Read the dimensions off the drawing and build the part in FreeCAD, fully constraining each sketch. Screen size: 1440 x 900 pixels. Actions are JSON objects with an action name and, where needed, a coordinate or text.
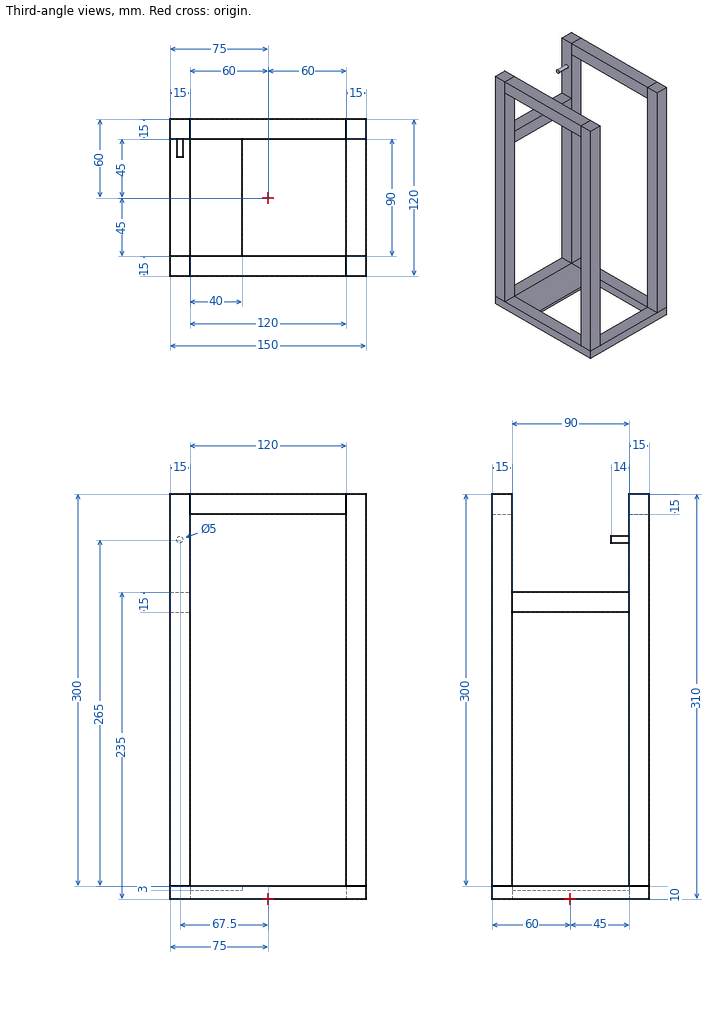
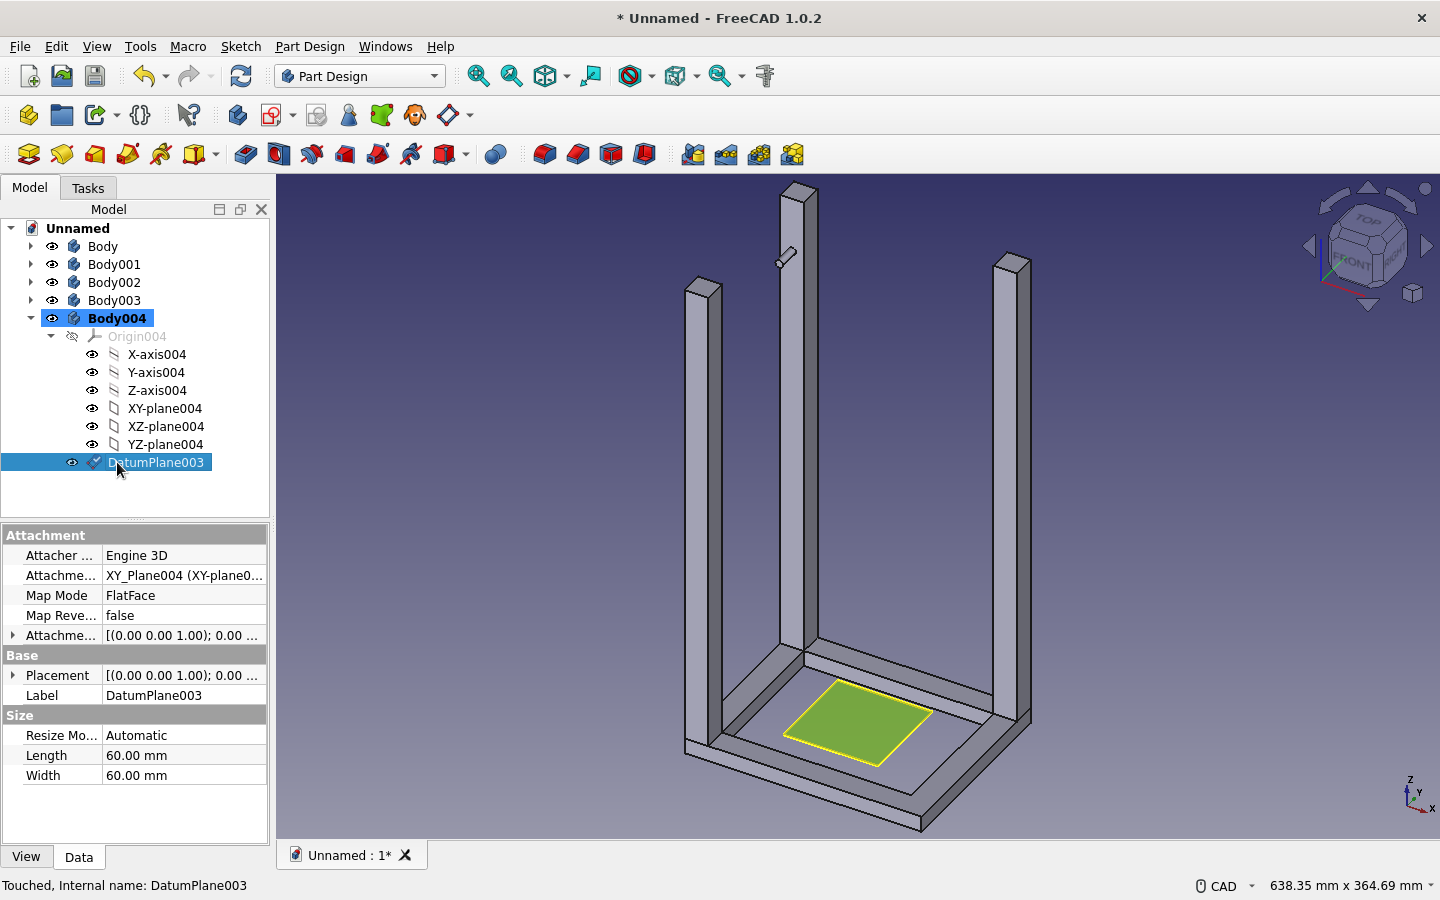
{"action": "left_click", "coordinate": [270, 116]}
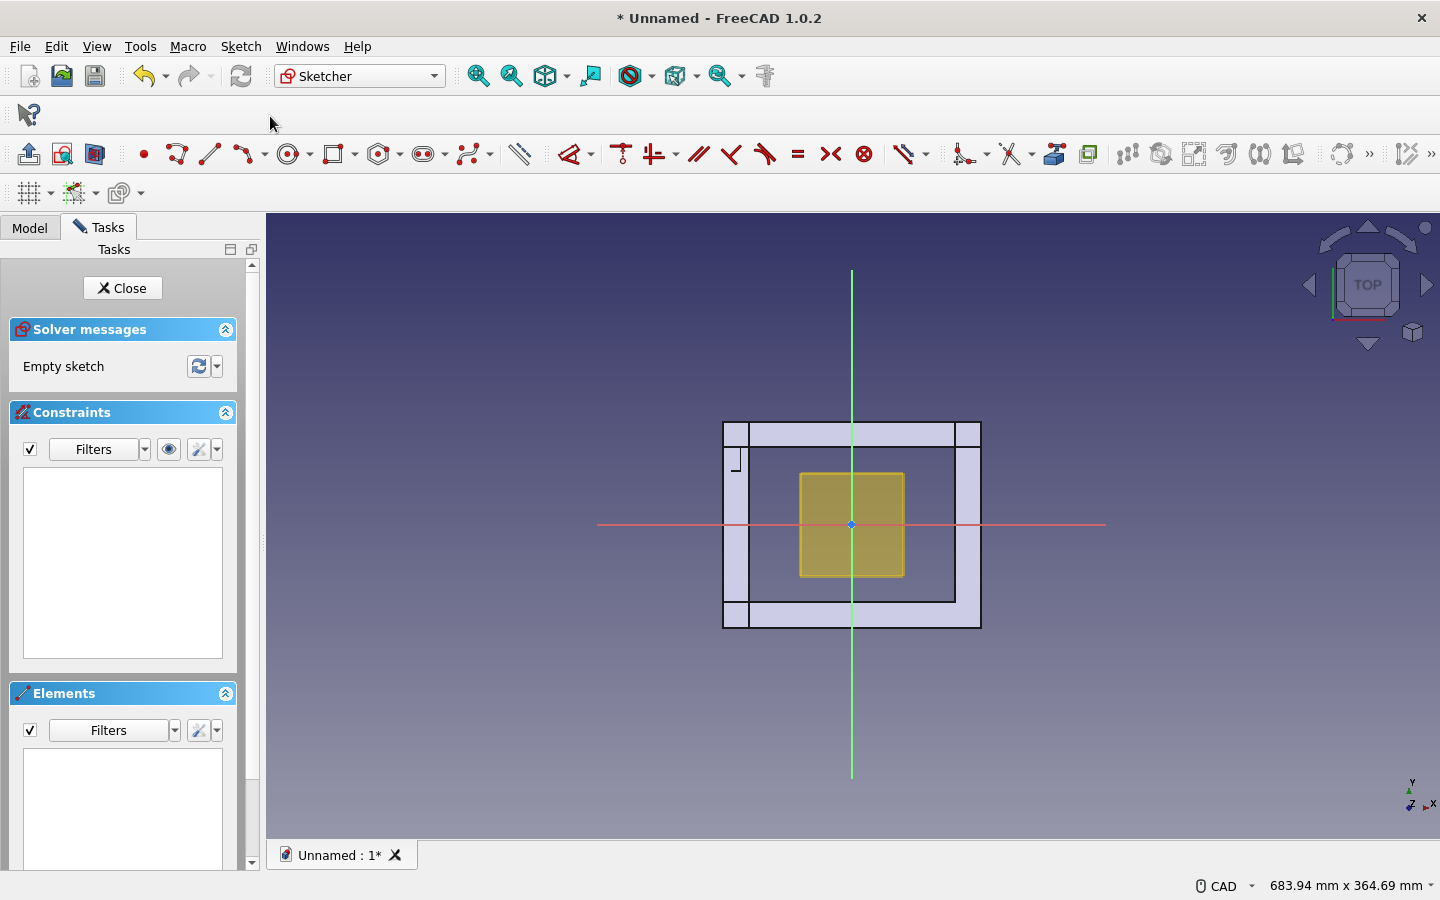
{"action": "scroll", "coordinate": [980, 620], "scroll_direction": "up", "scroll_amount": 14}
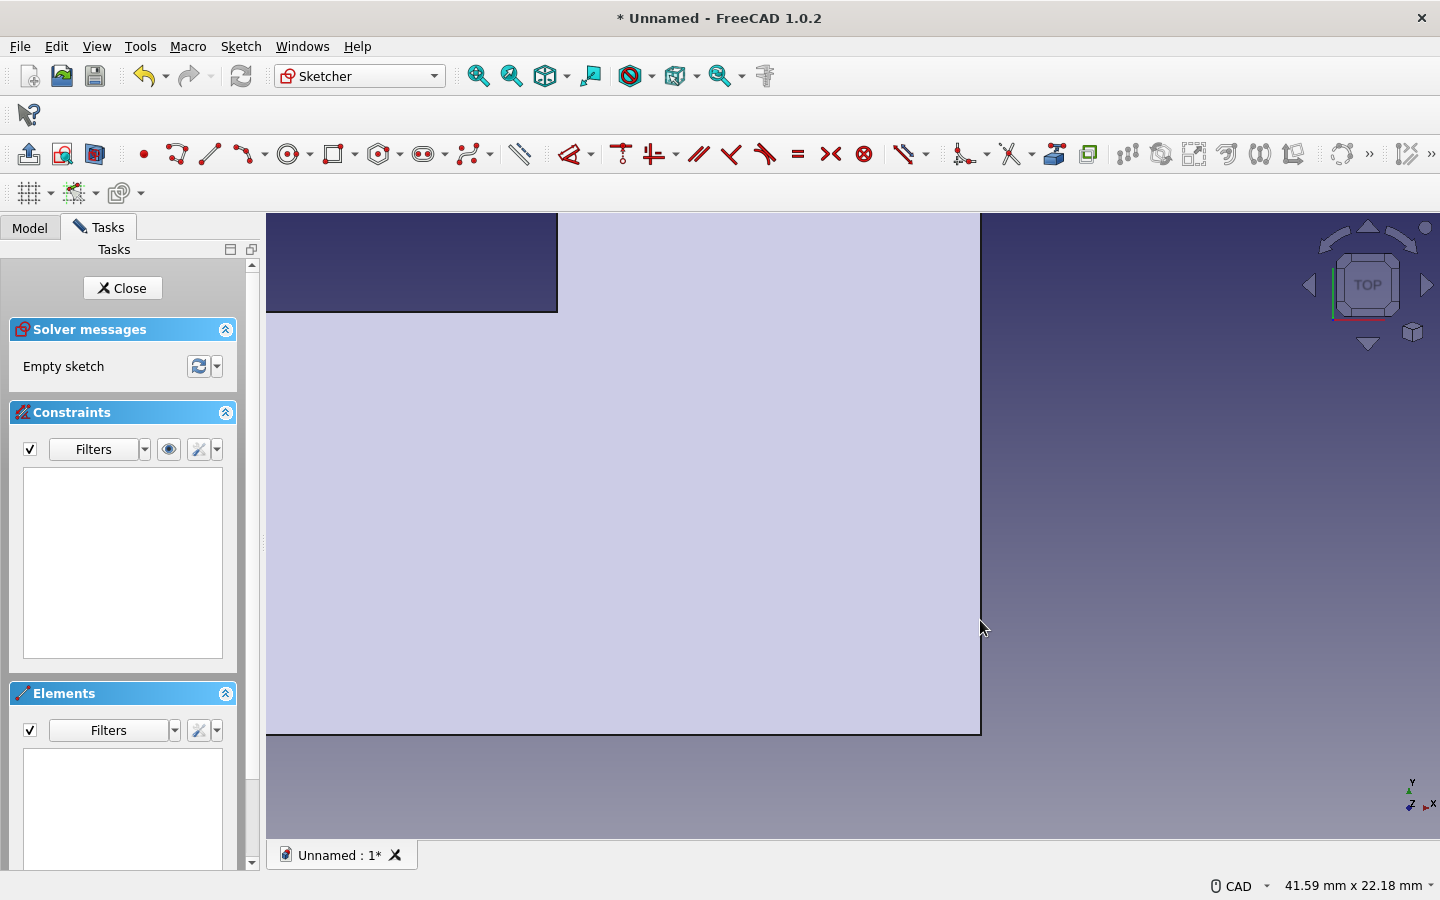
{"action": "left_click", "coordinate": [332, 154]}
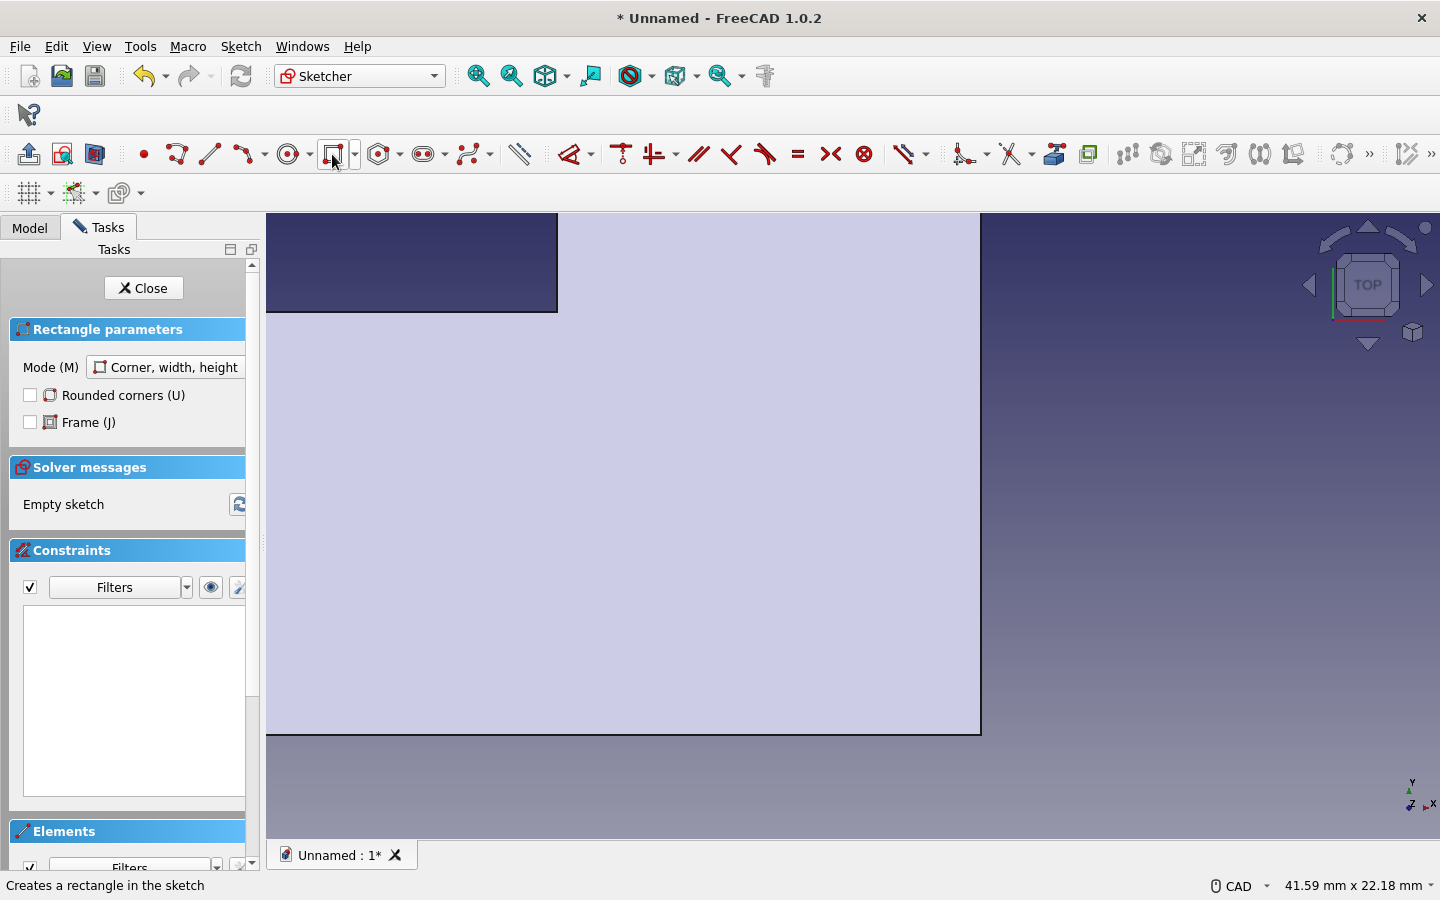
{"action": "left_click", "coordinate": [557, 312]}
{"action": "left_click", "coordinate": [981, 735]}
{"action": "key", "text": "Escape"}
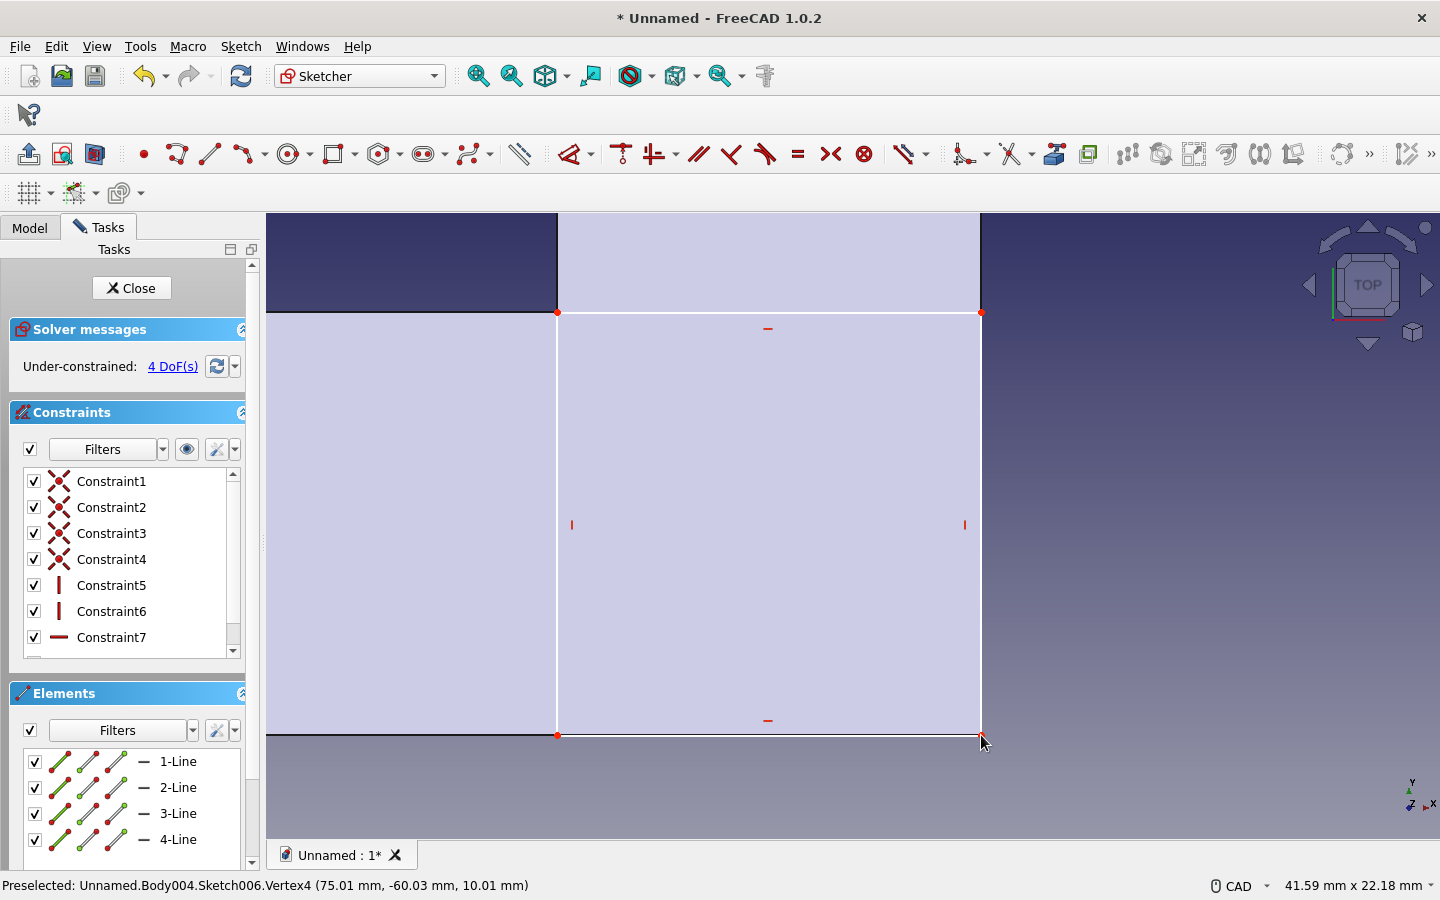
{"action": "left_click", "coordinate": [568, 154]}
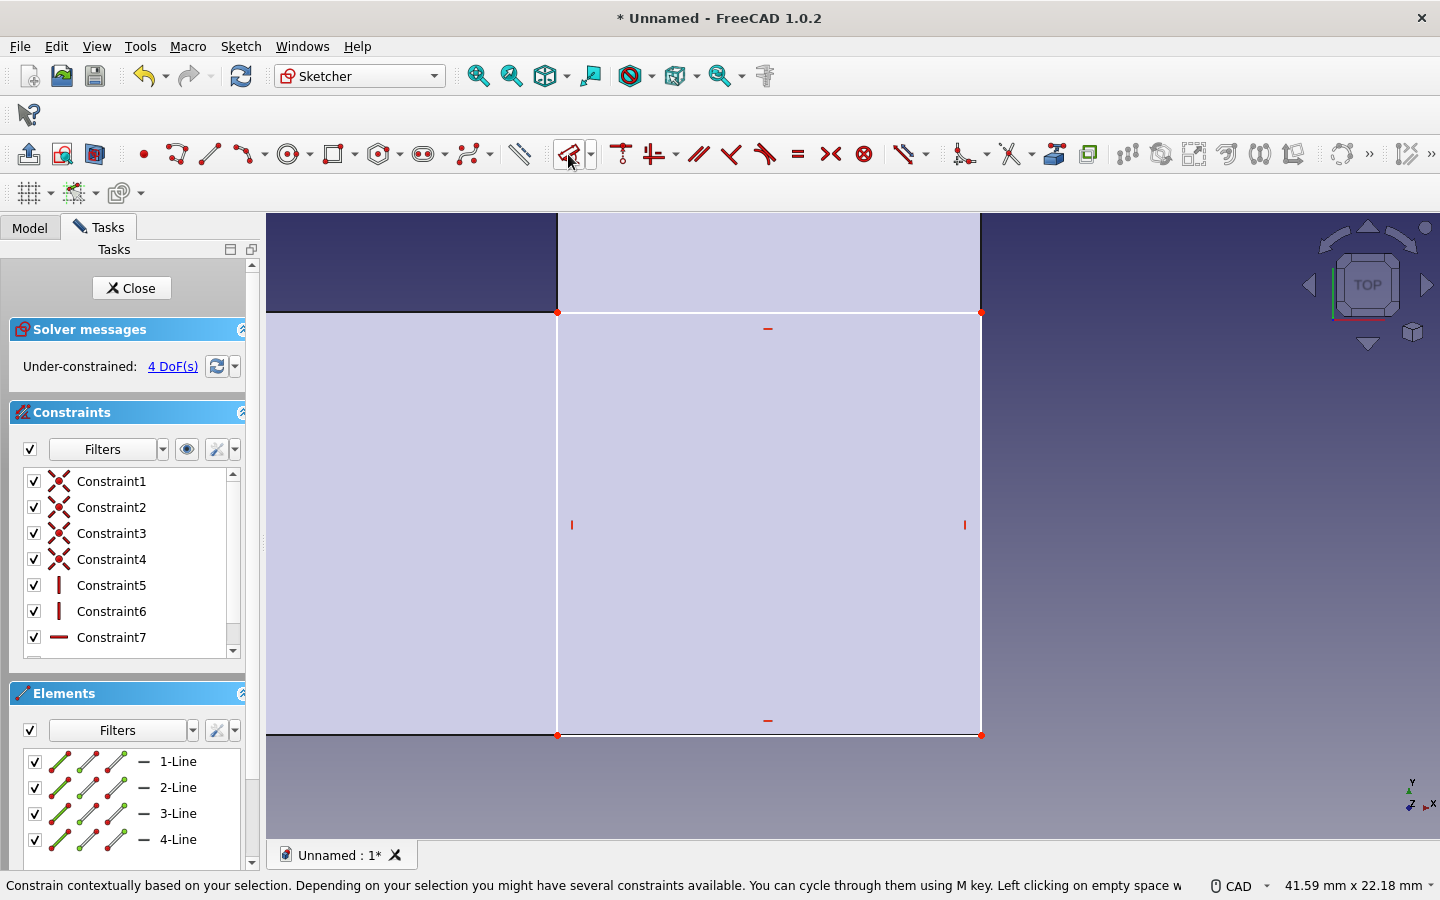
{"action": "left_click", "coordinate": [557, 440]}
{"action": "left_click", "coordinate": [523, 524]}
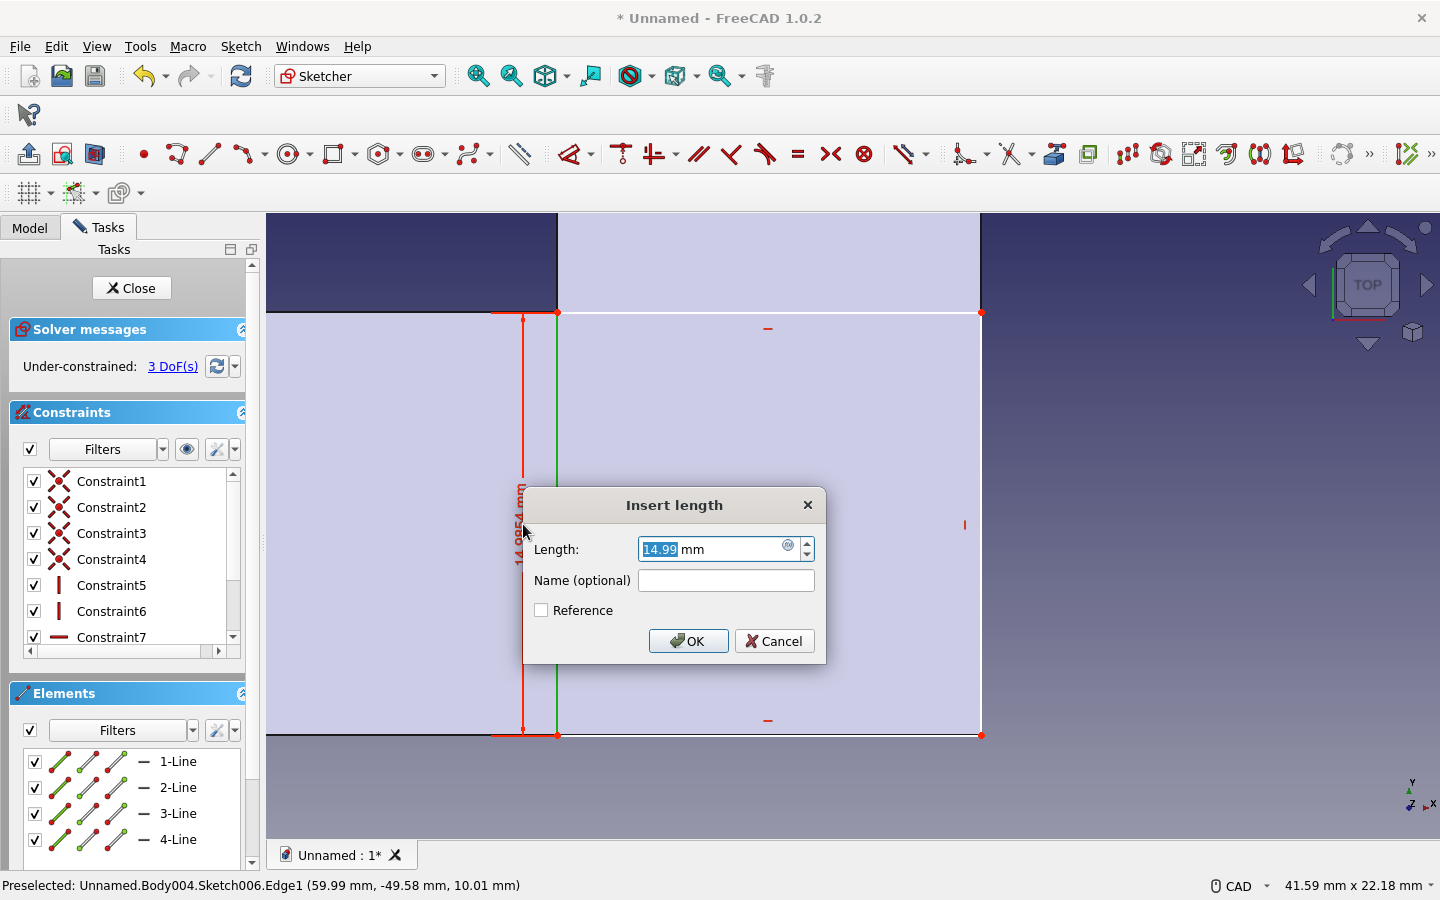
{"action": "type", "text": "15"}
{"action": "key", "text": "Return"}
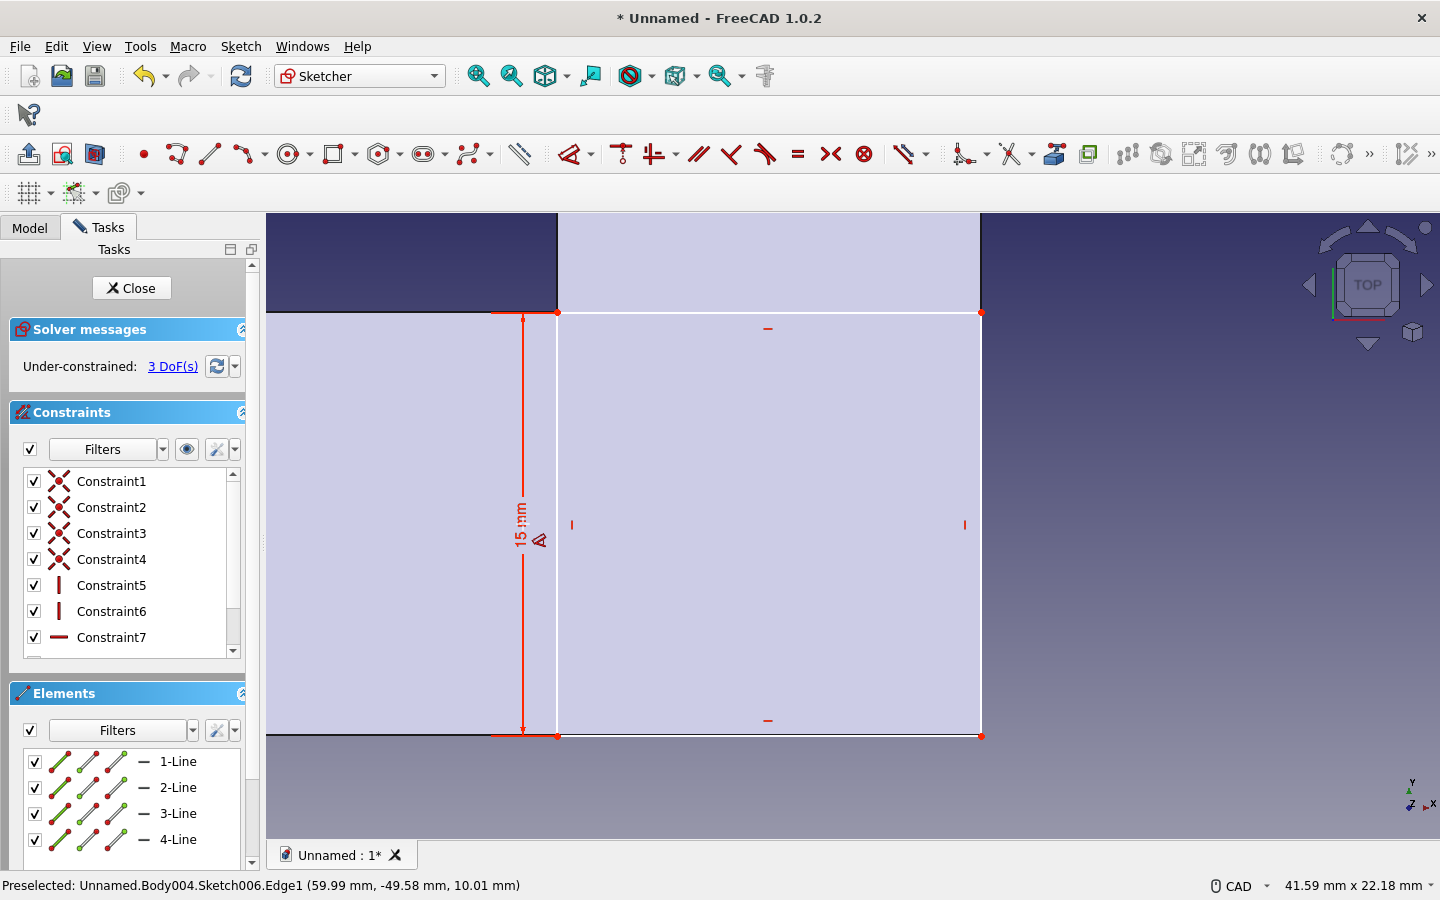
{"action": "left_click", "coordinate": [684, 736]}
{"action": "left_click", "coordinate": [769, 770]}